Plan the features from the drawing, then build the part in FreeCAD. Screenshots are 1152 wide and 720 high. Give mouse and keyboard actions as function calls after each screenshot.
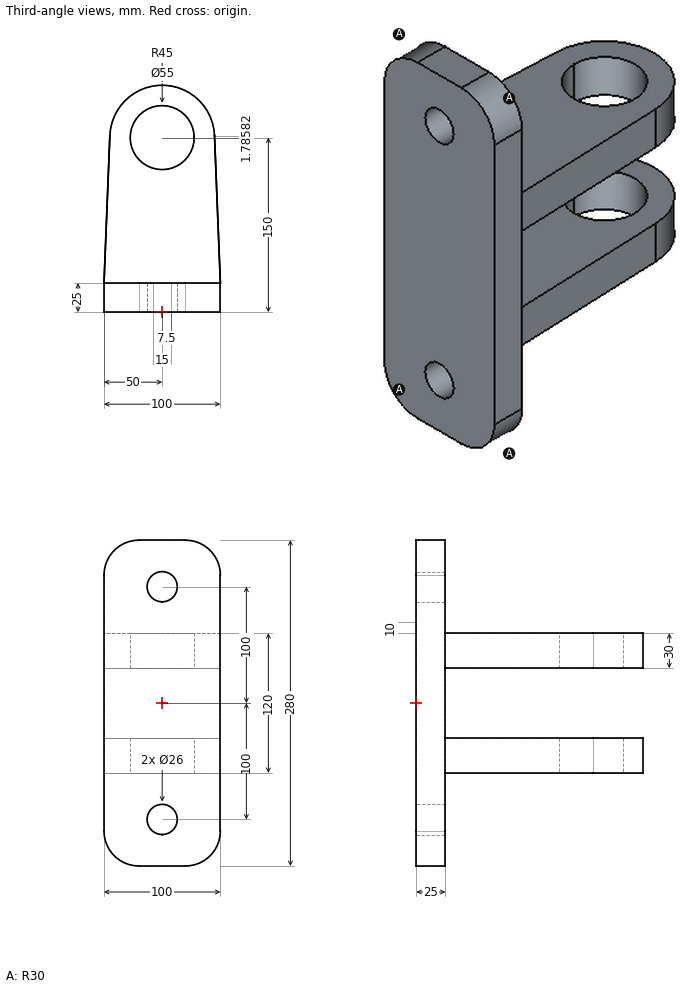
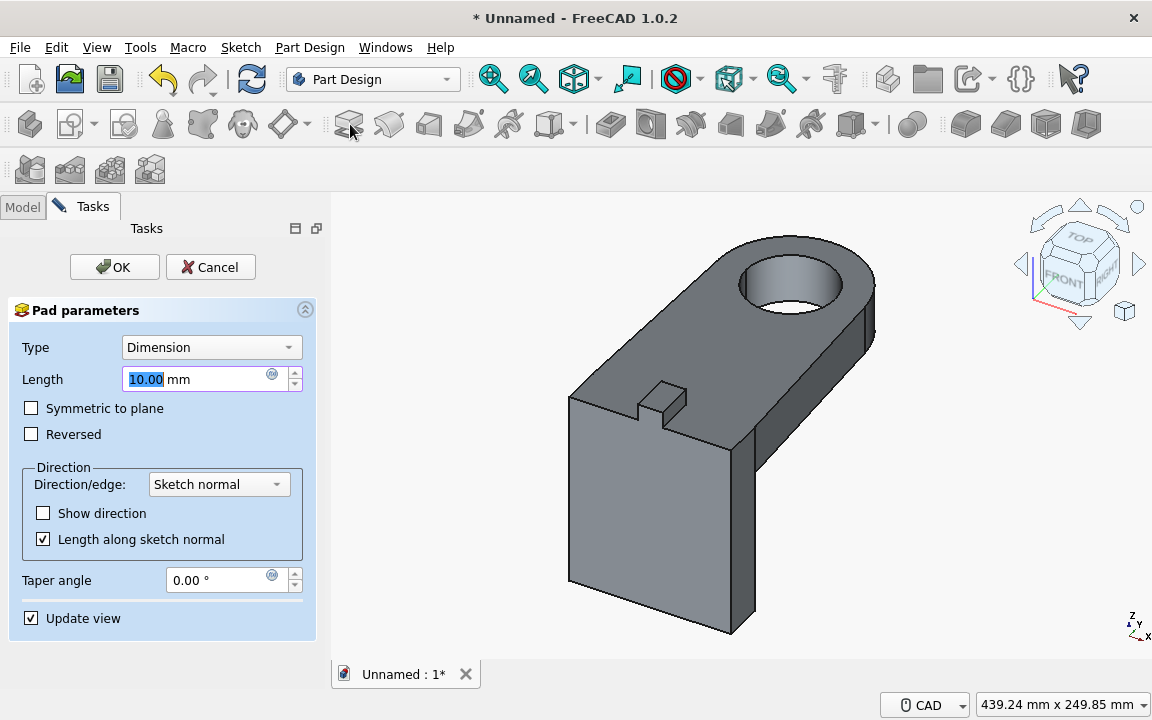
text(10)
key(Tab)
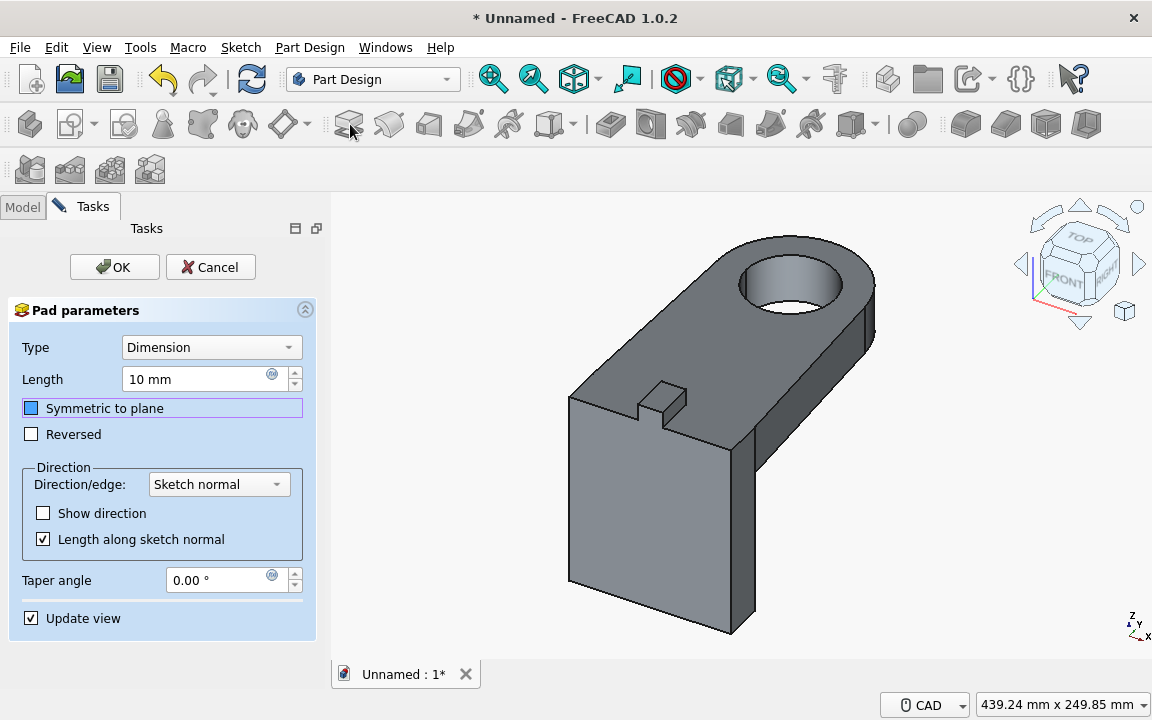
click(115, 267)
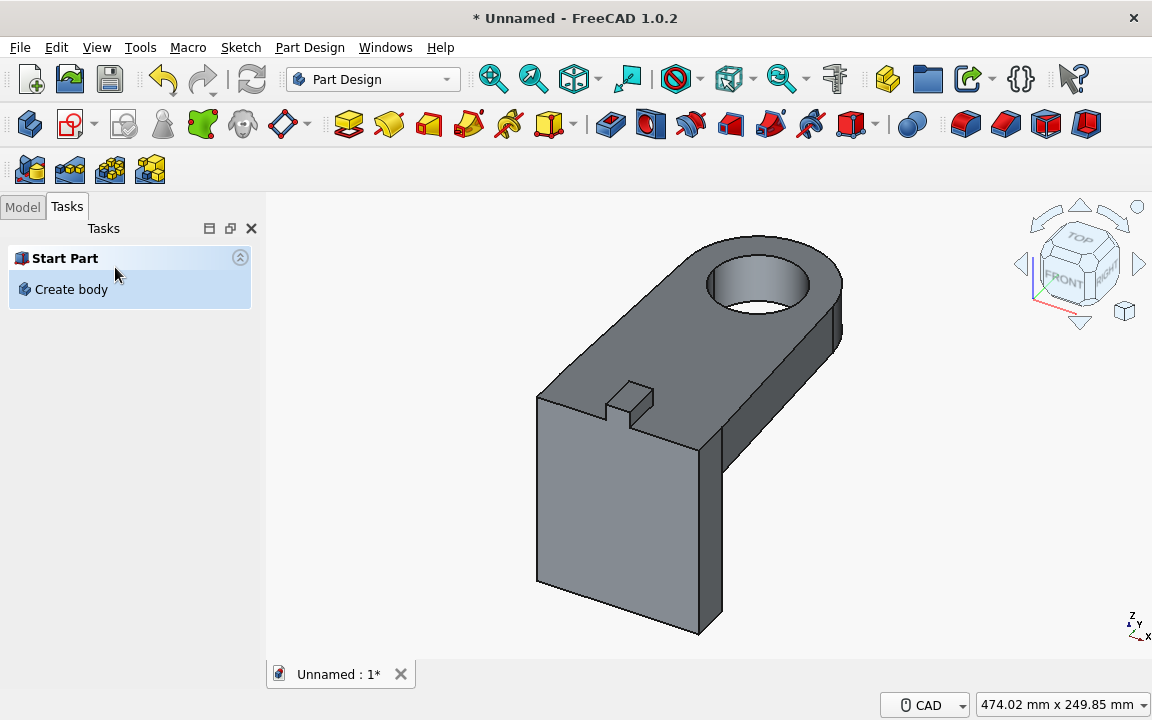
click(23, 206)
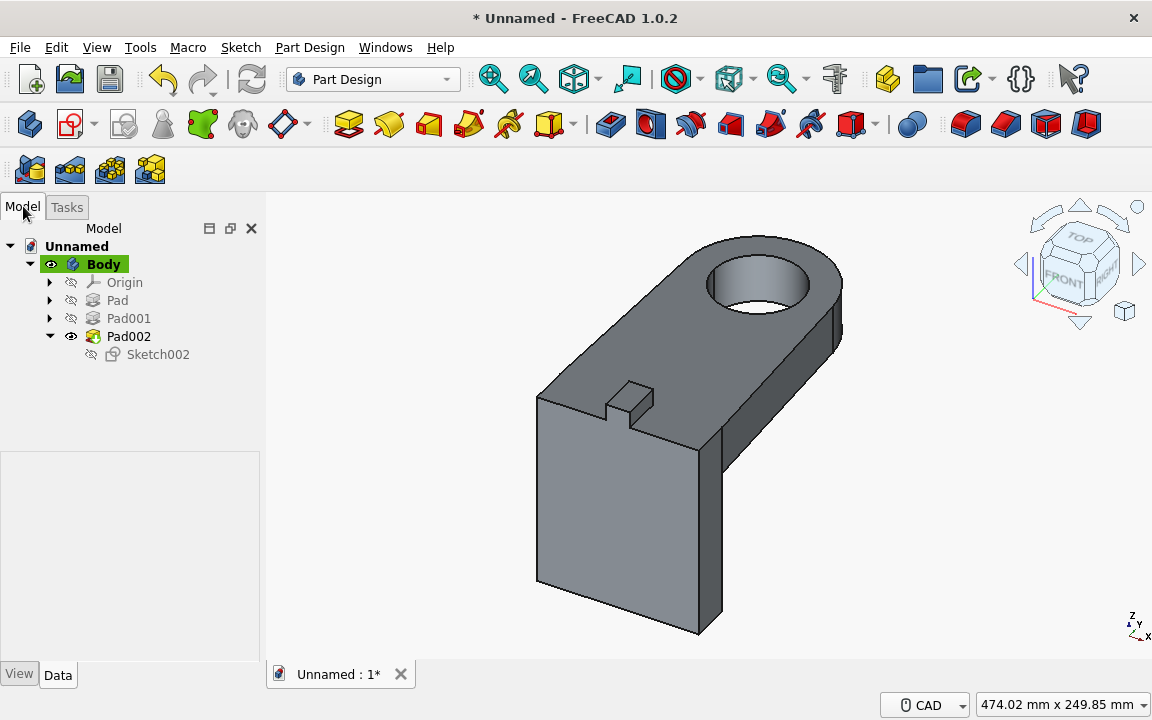
click(116, 318)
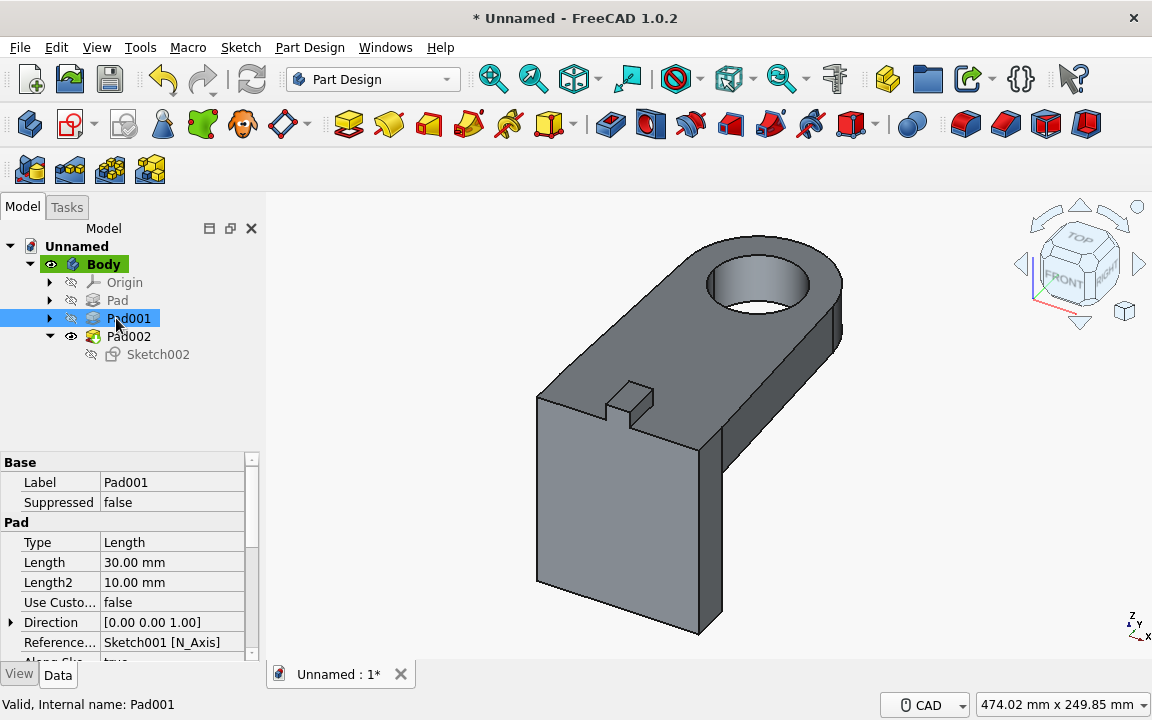
click(116, 336, ctrl)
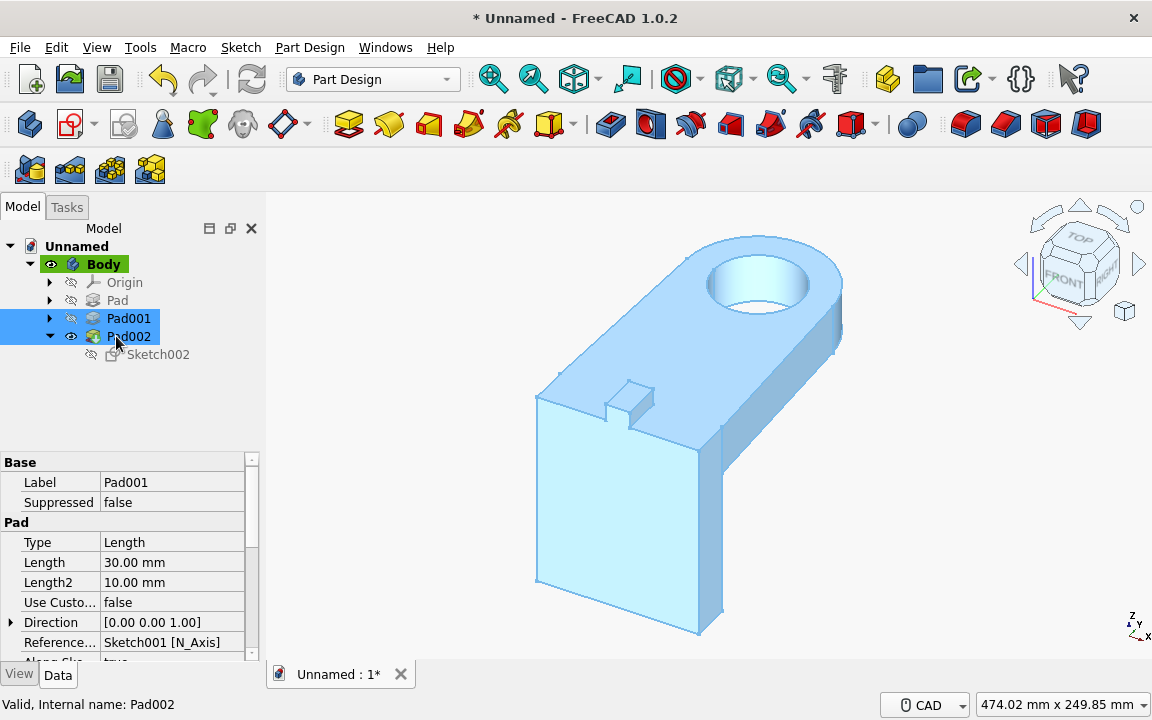
click(30, 170)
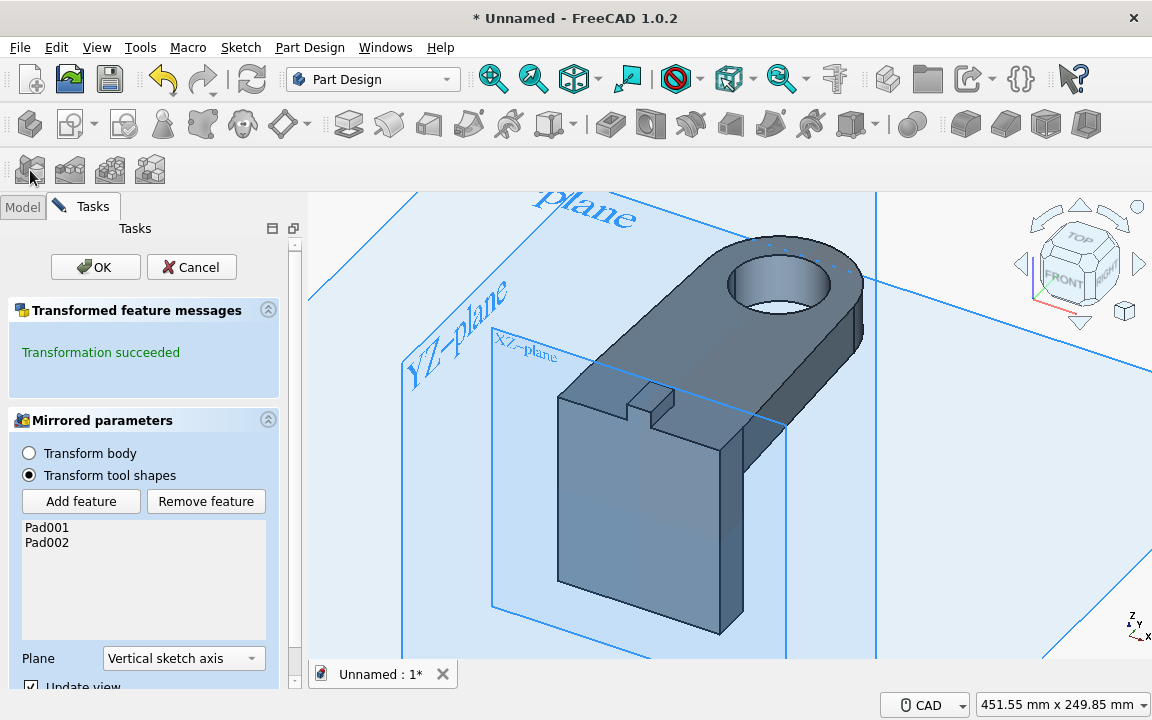
click(184, 658)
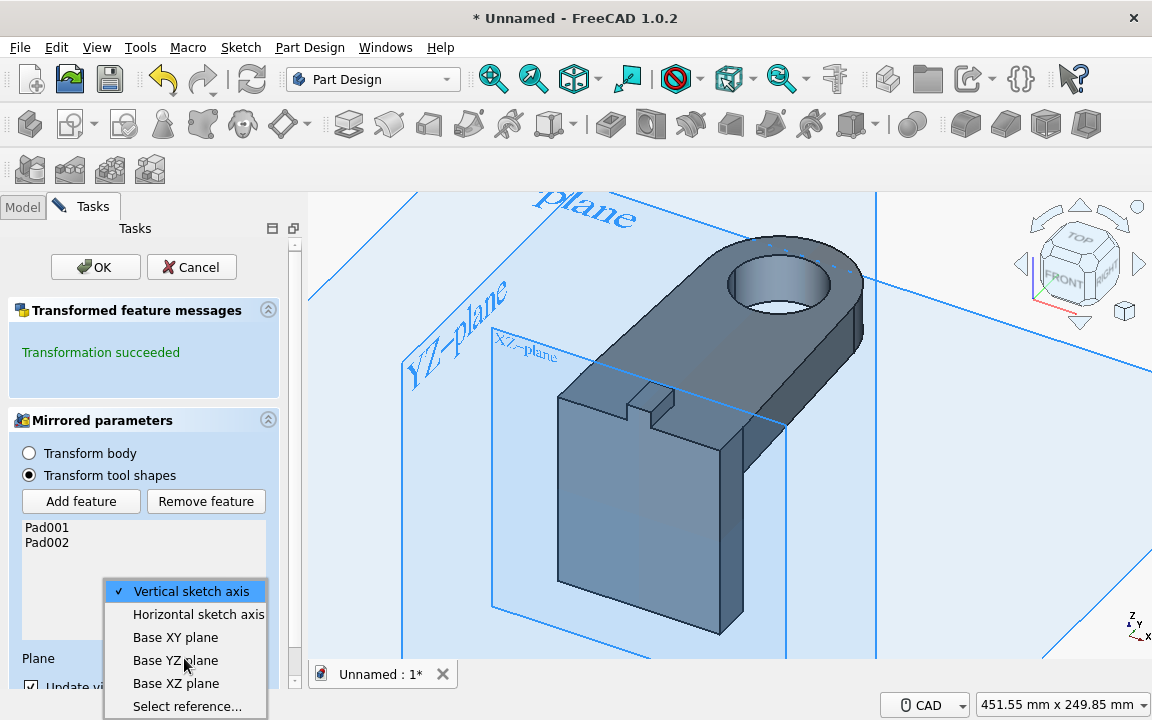
click(184, 638)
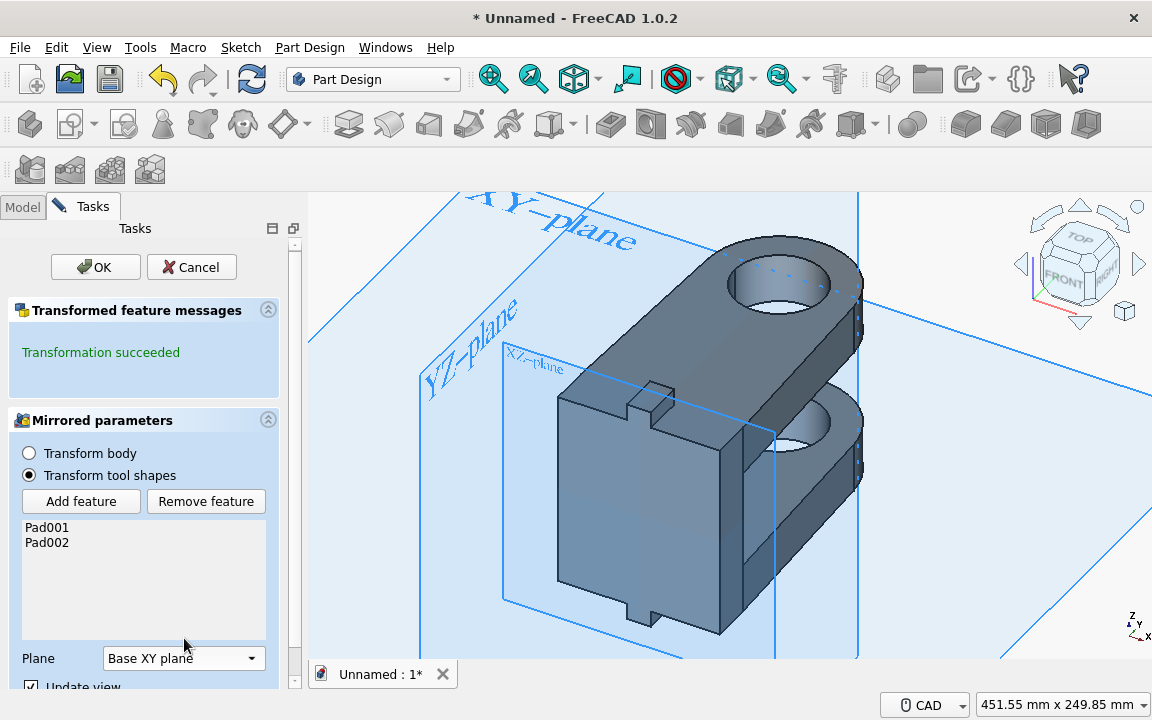
click(96, 267)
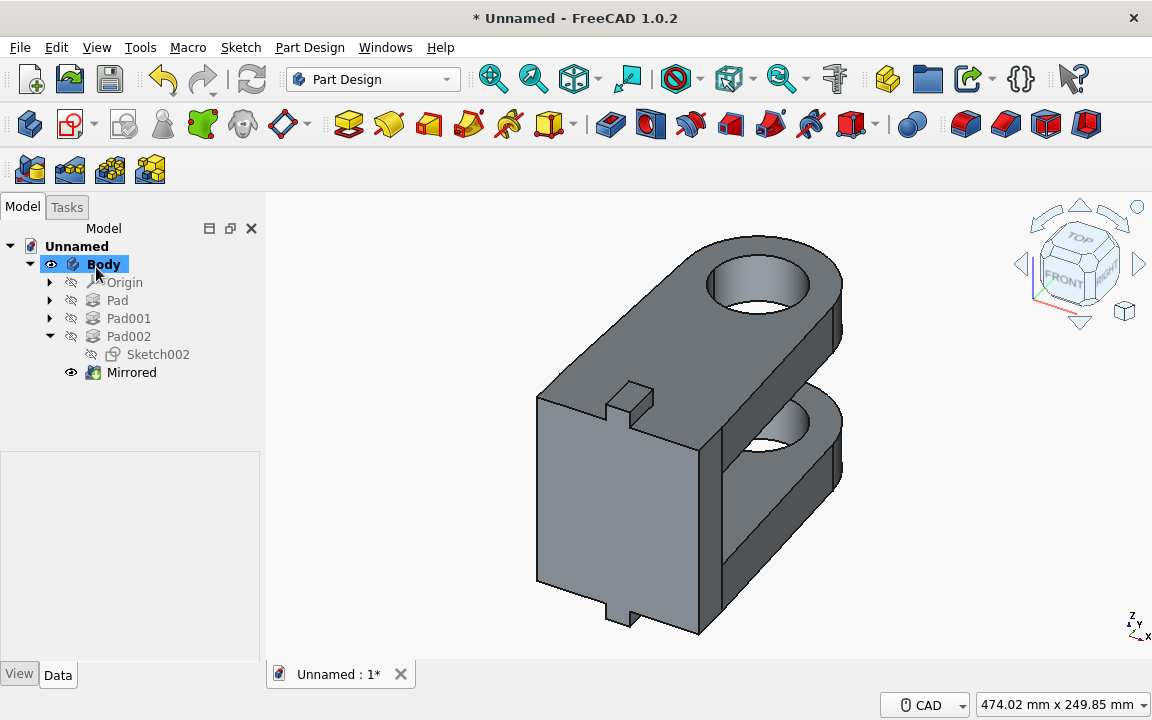
click(70, 124)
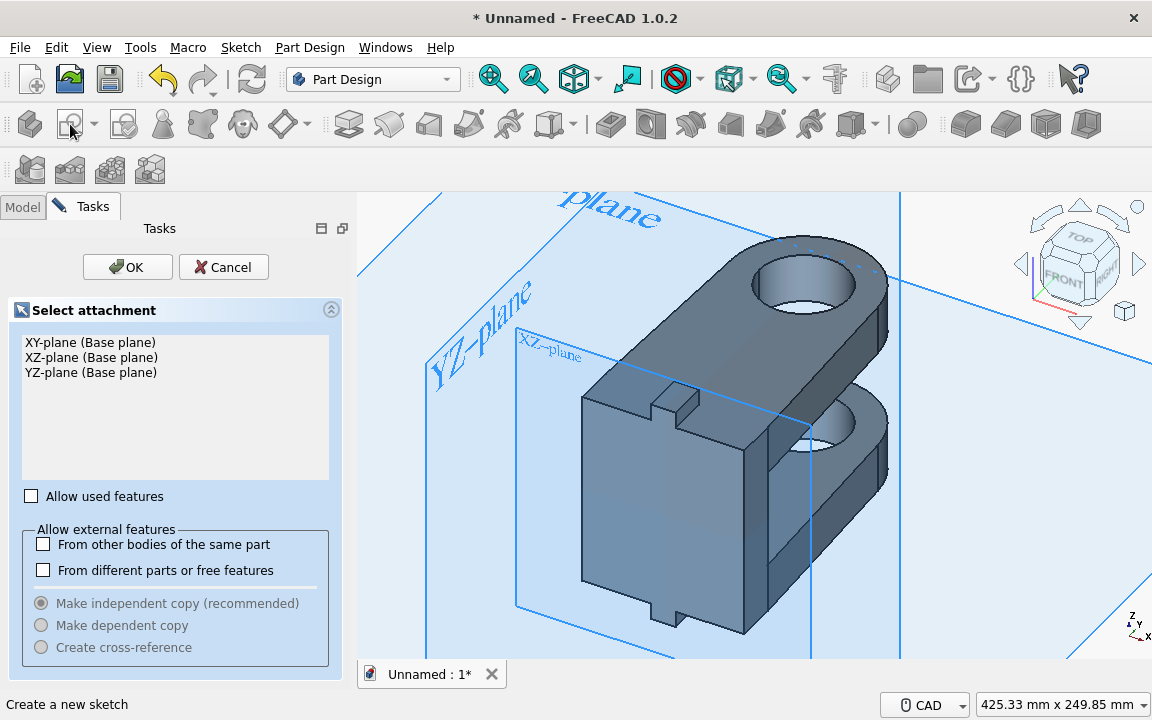
click(82, 358)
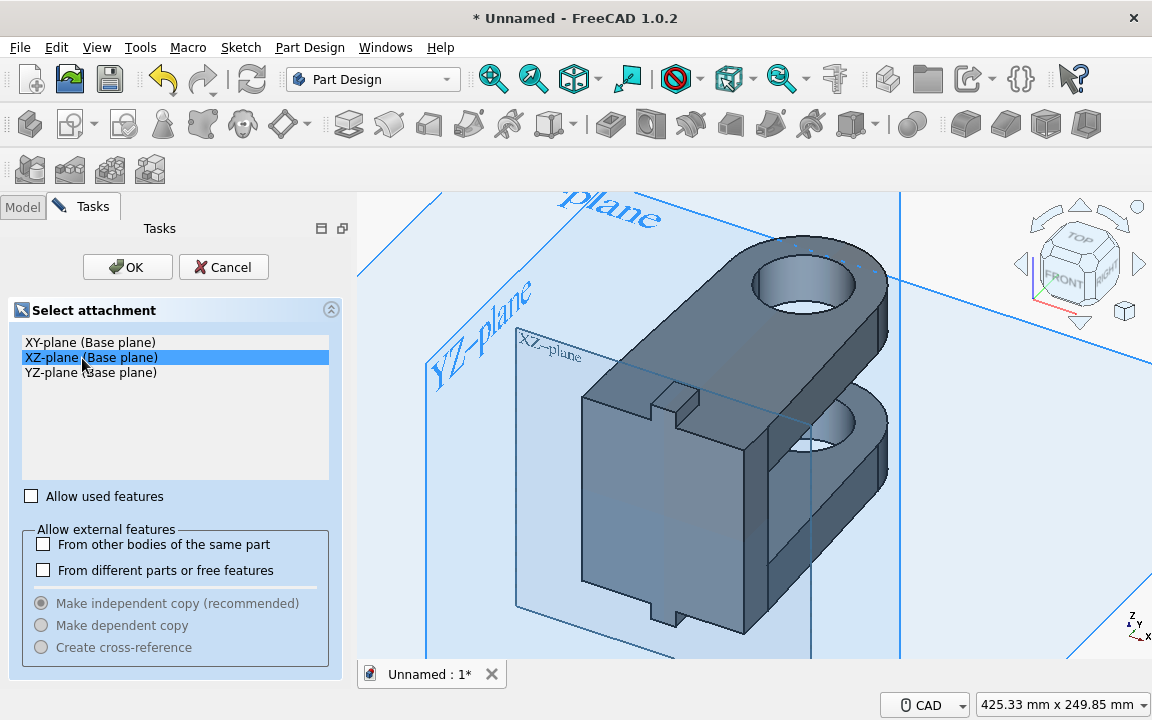
click(128, 267)